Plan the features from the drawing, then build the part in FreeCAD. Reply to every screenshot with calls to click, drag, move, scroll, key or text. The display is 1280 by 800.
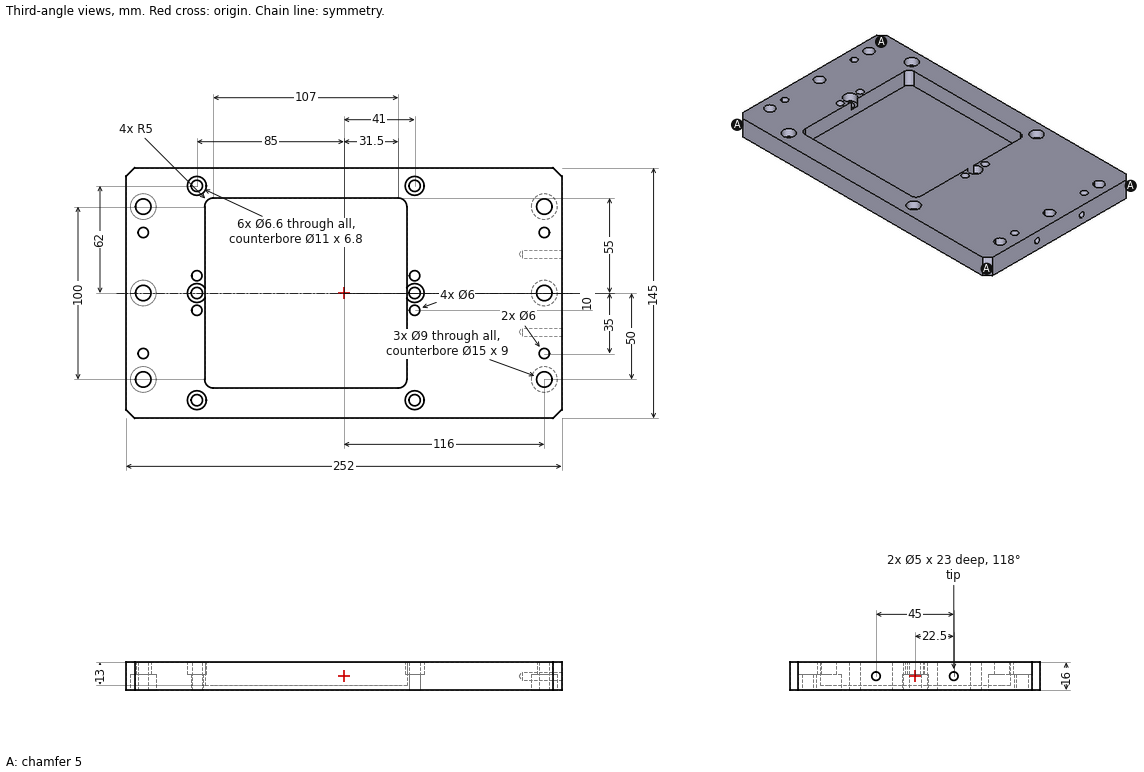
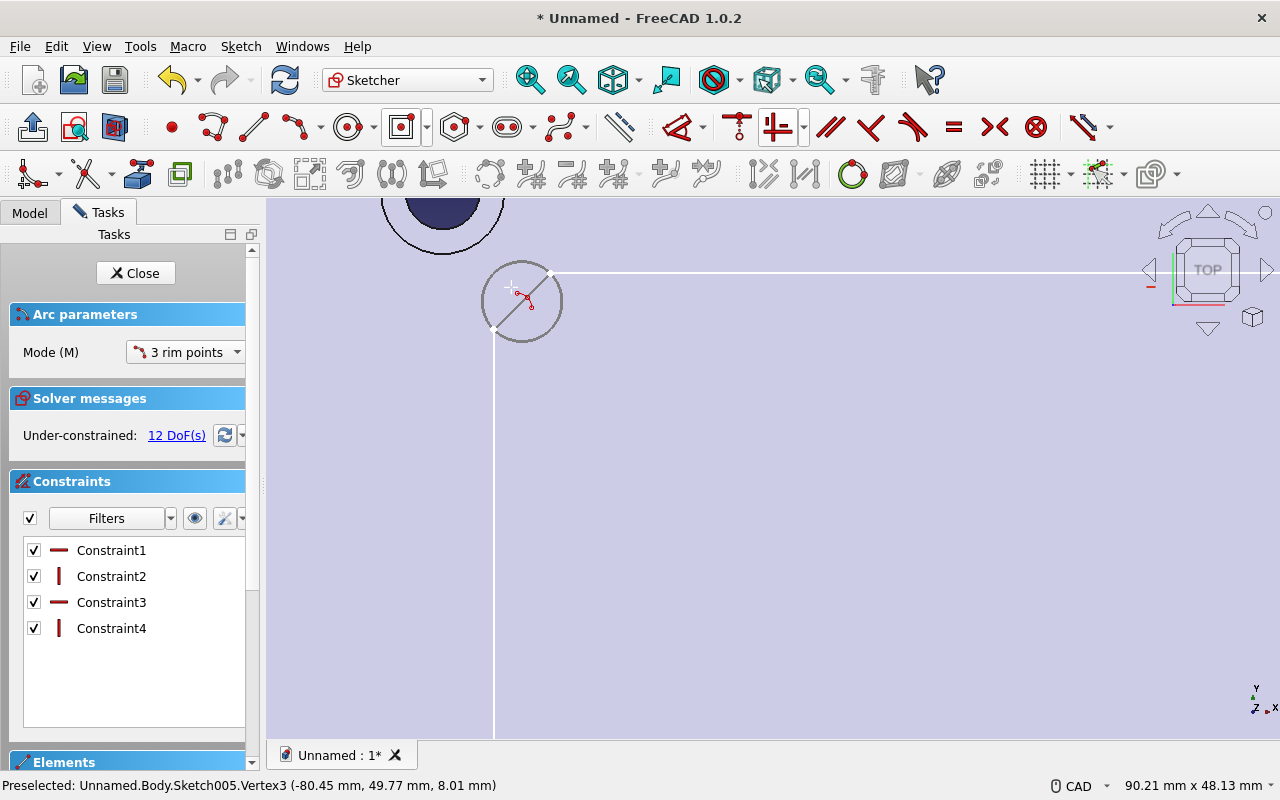
click(510, 287)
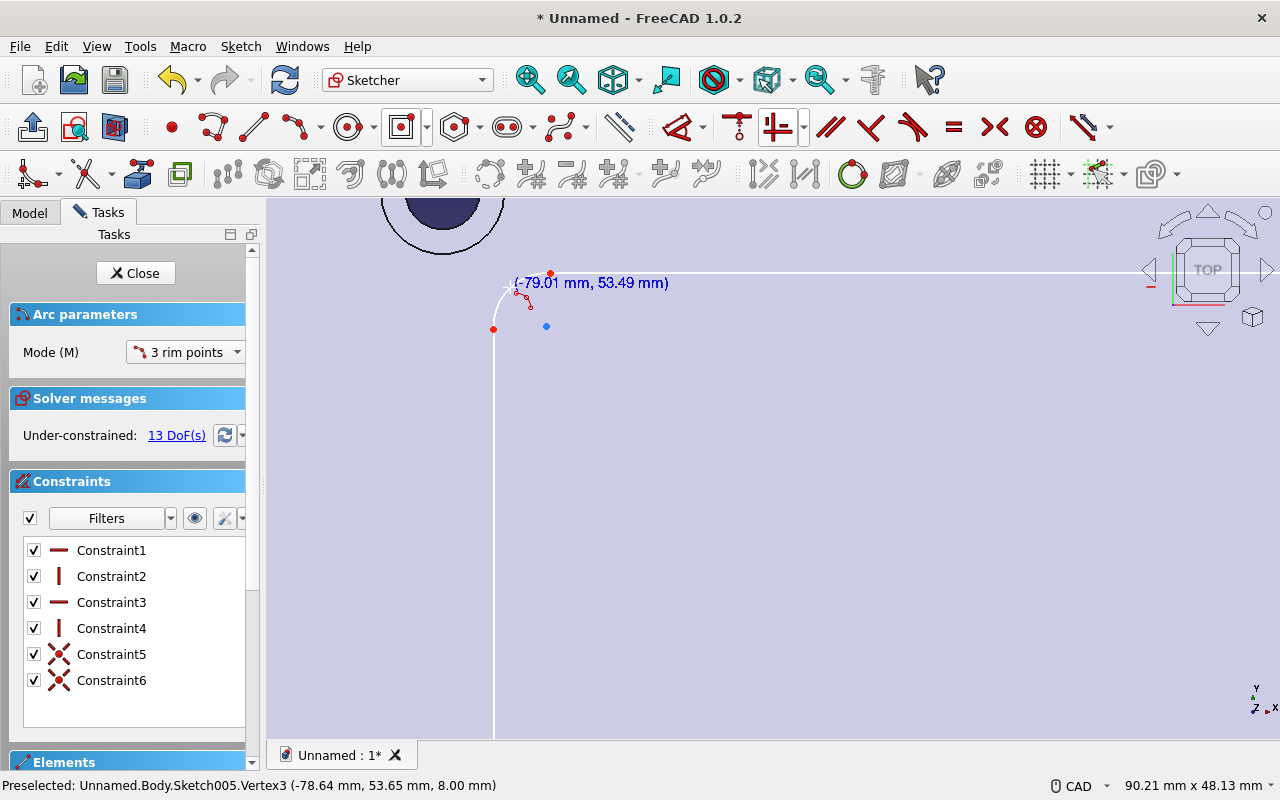
scroll(512, 287, down, 6)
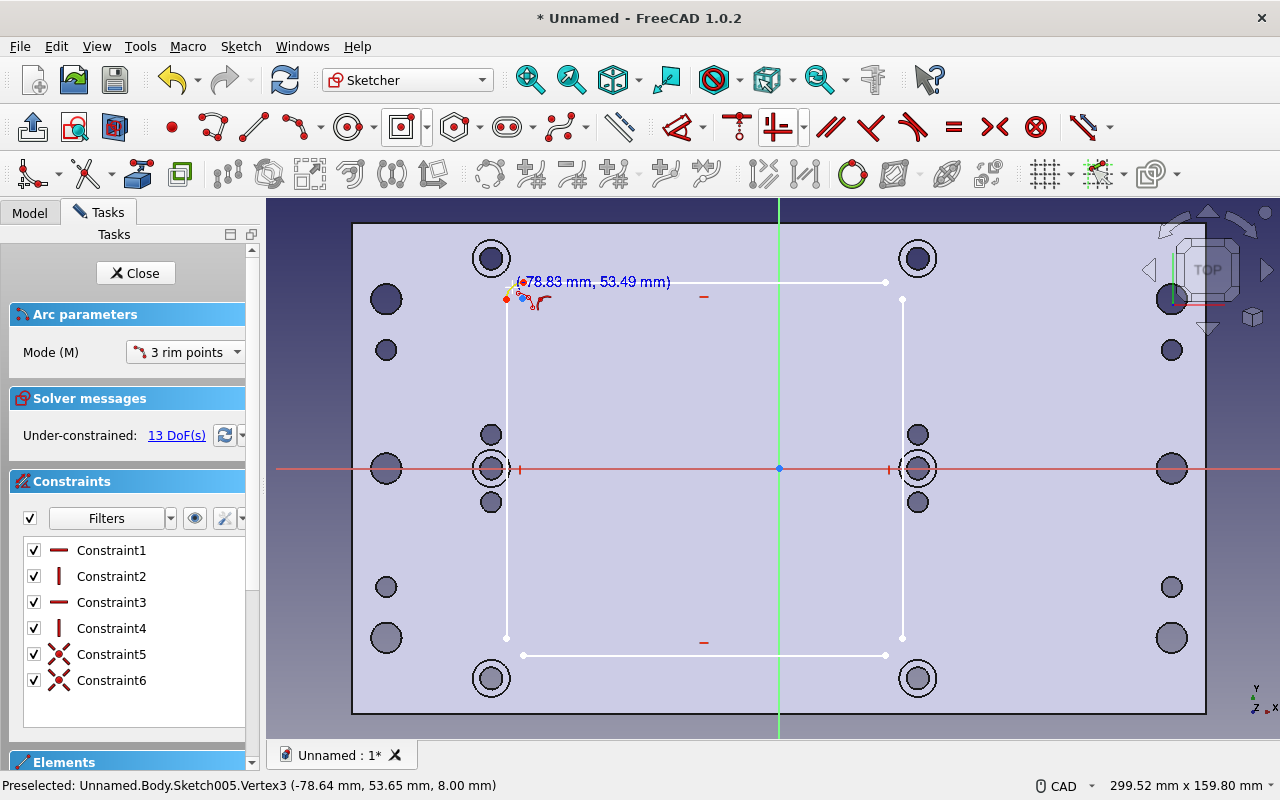
click(507, 639)
click(524, 656)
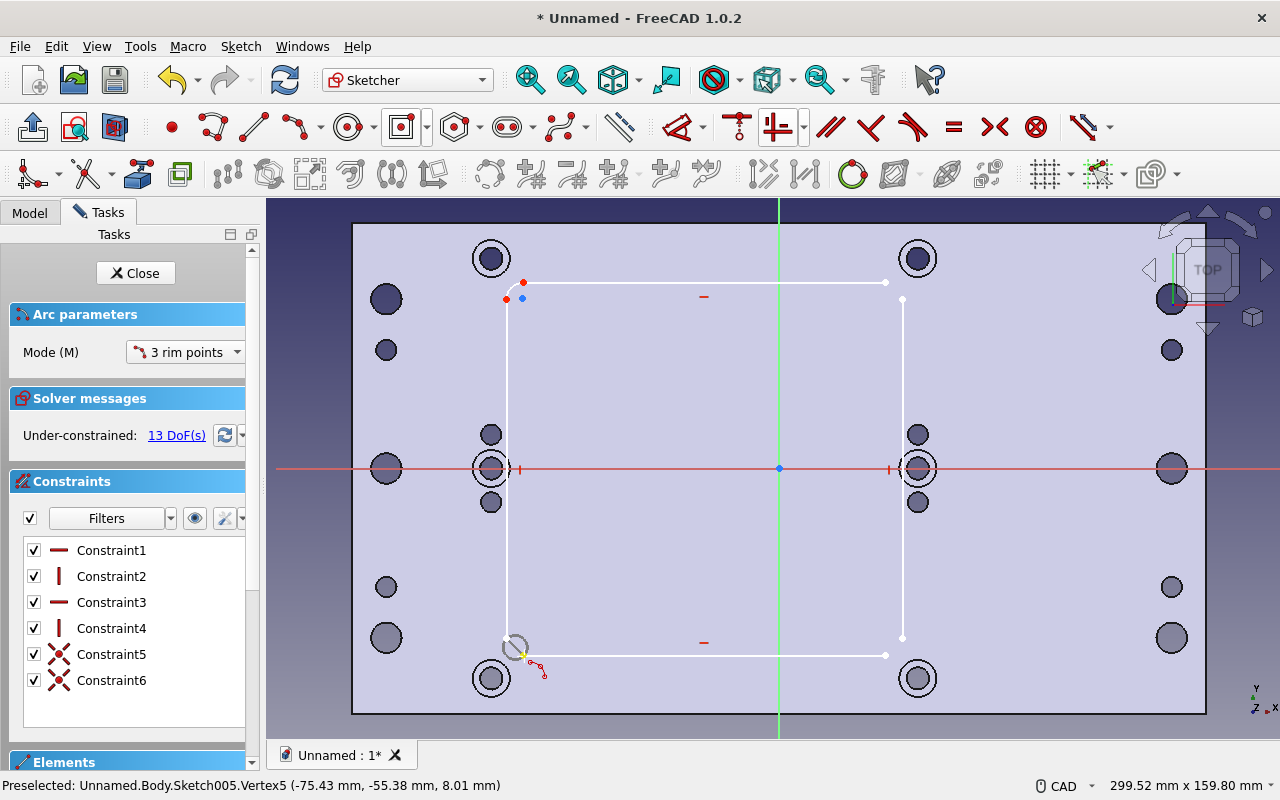
scroll(511, 650, up, 6)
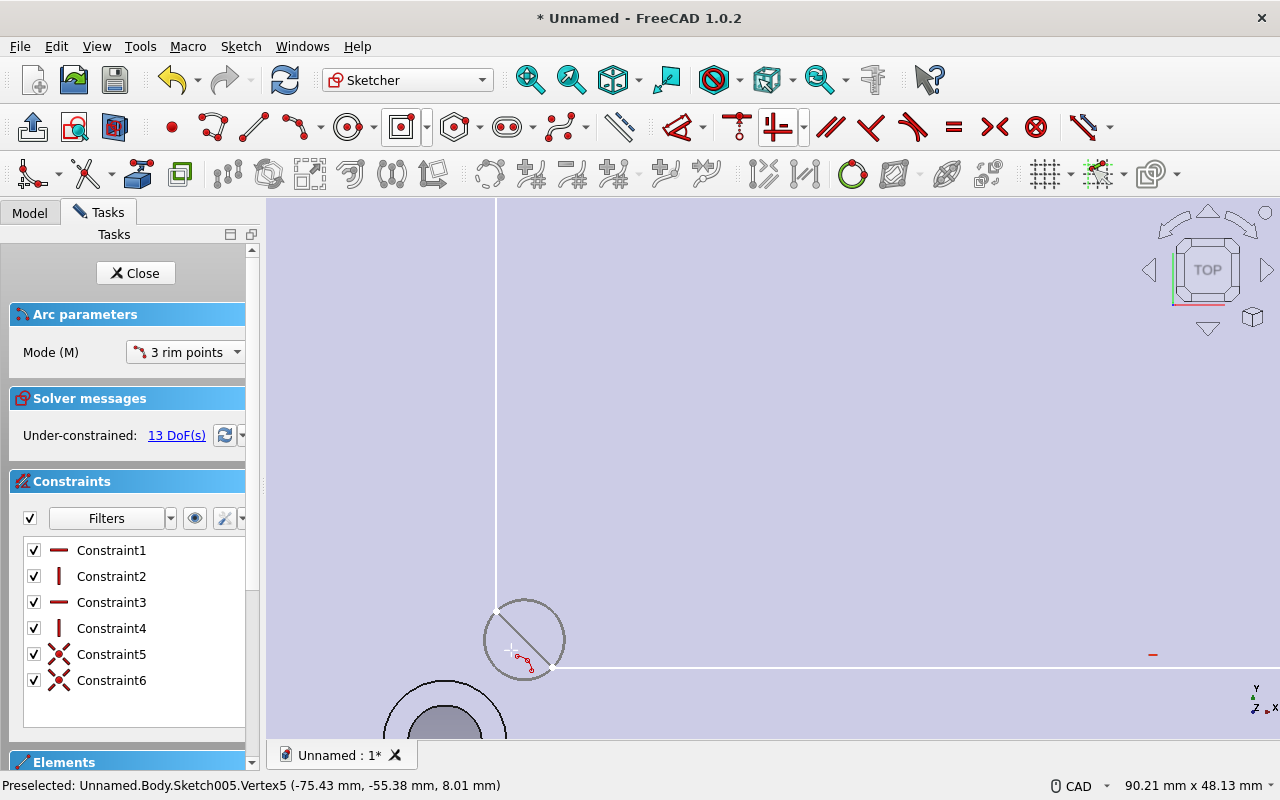
click(512, 647)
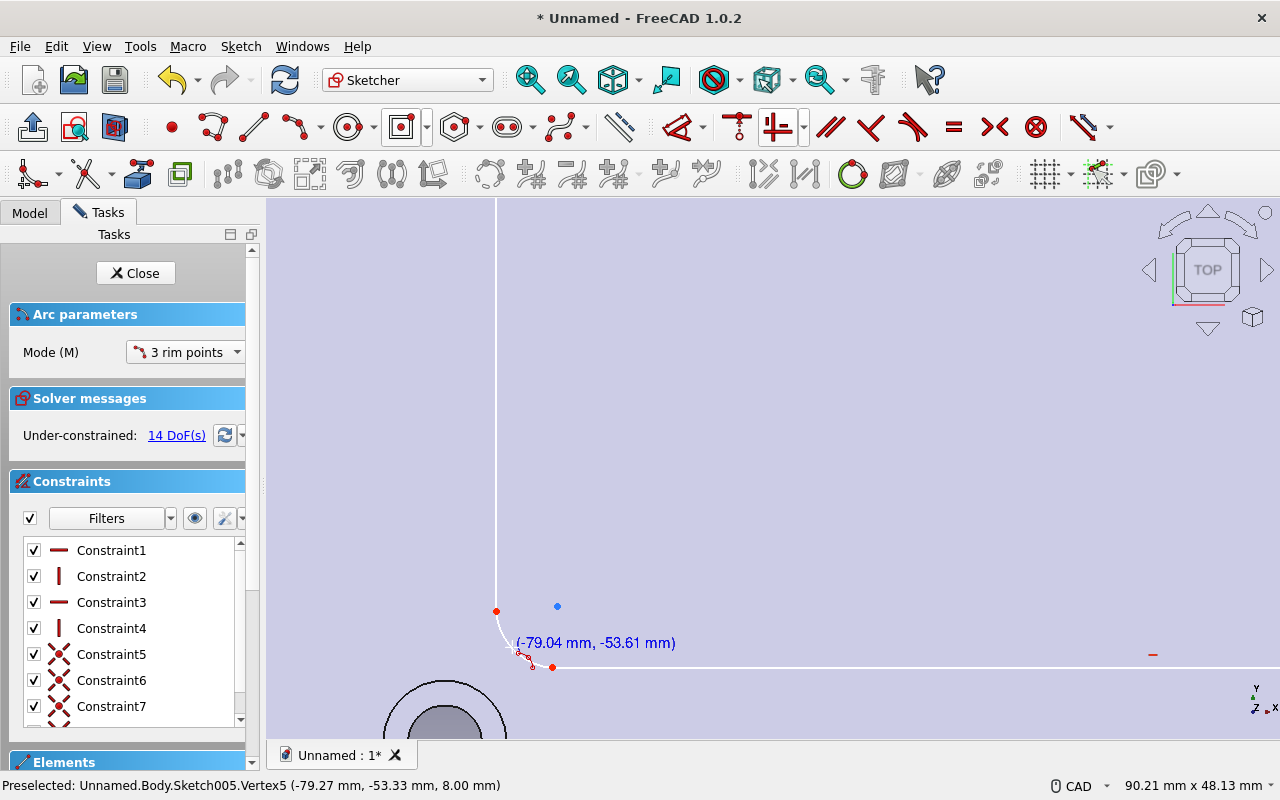
scroll(511, 651, down, 6)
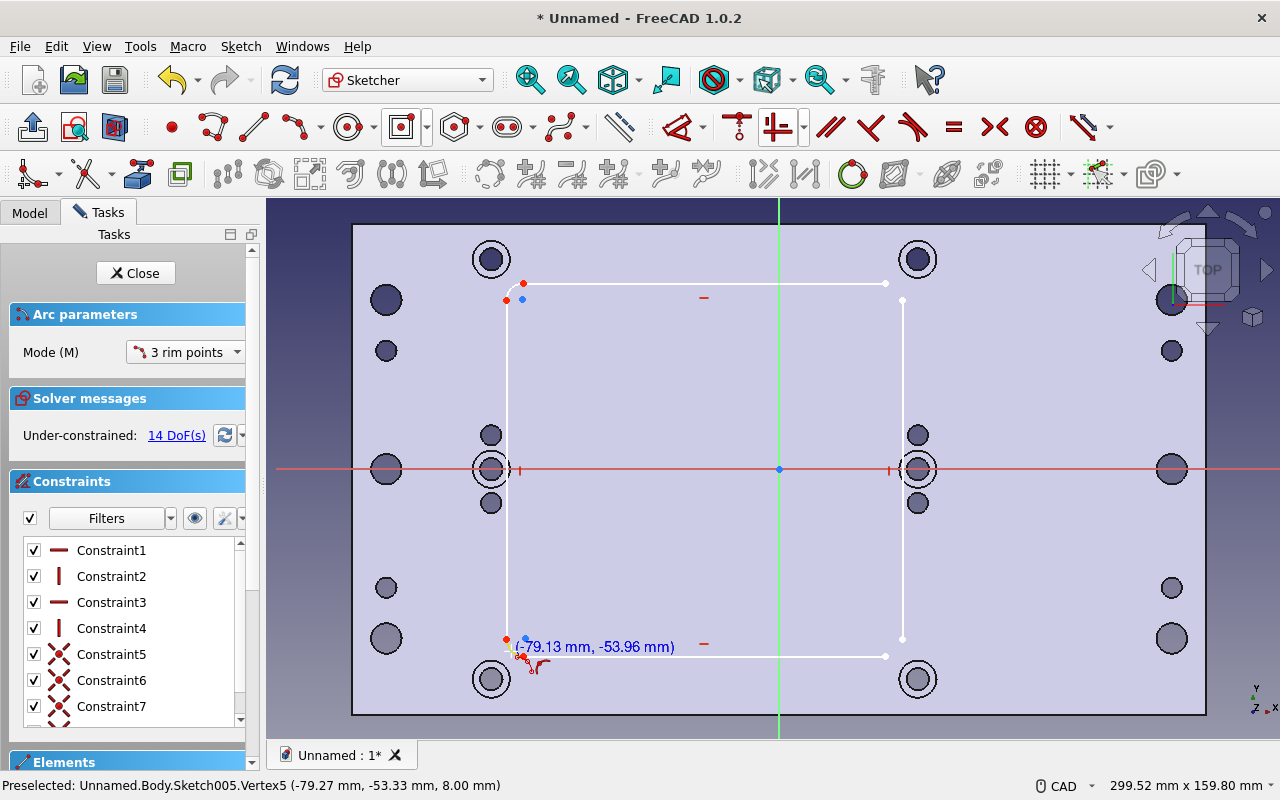
click(886, 657)
click(903, 640)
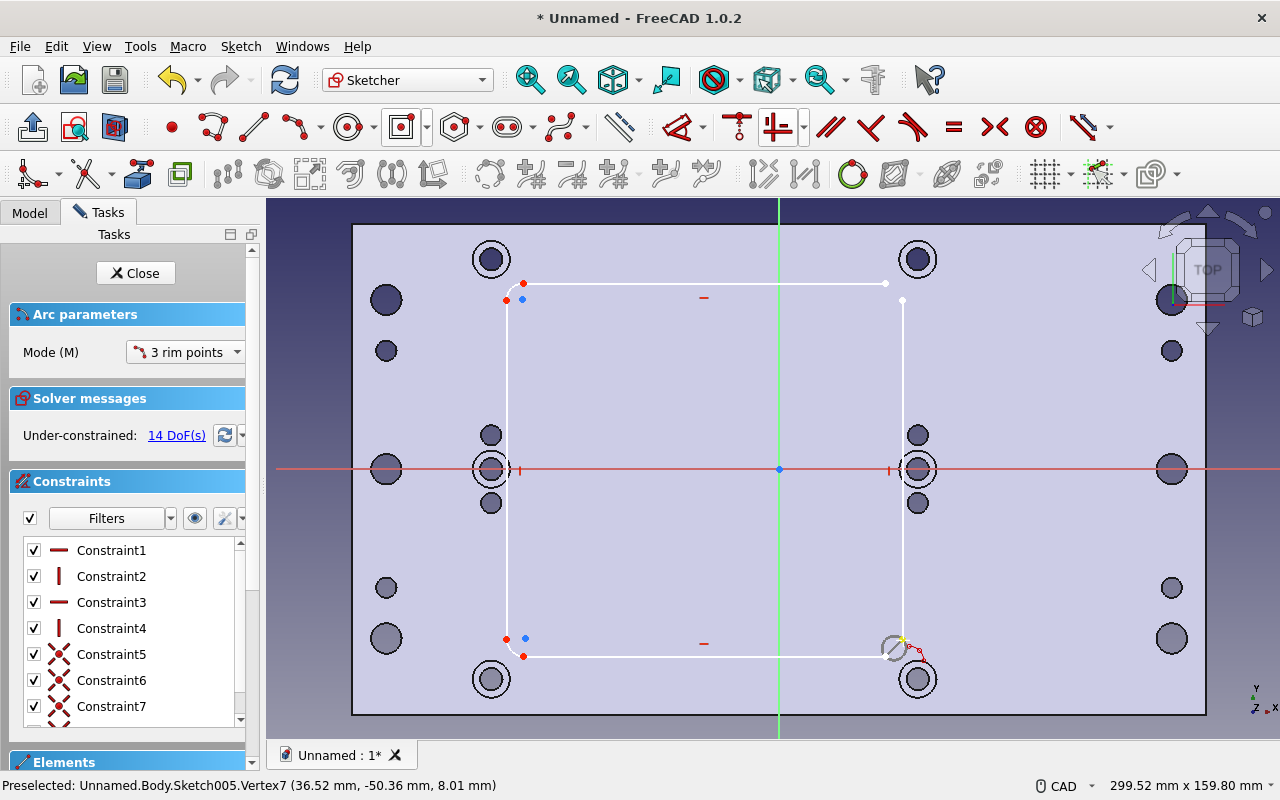
scroll(898, 650, up, 6)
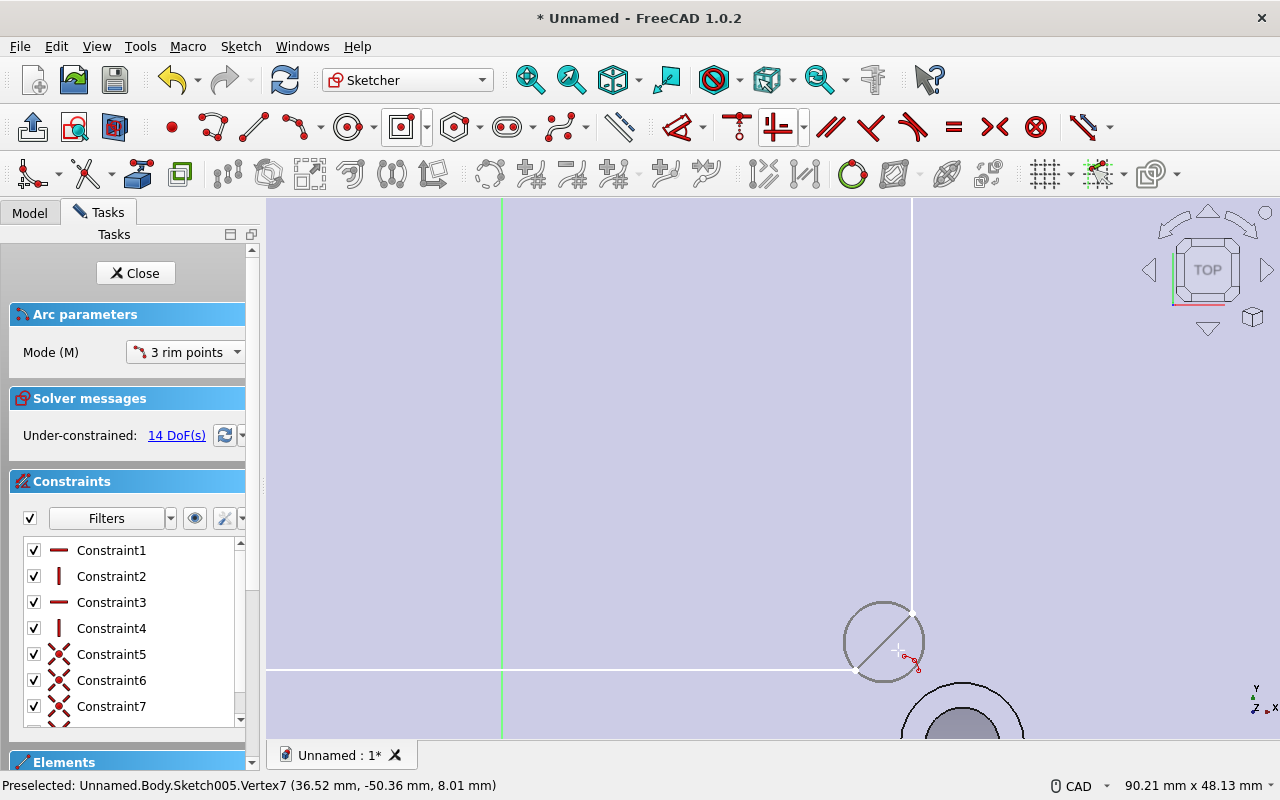
click(895, 650)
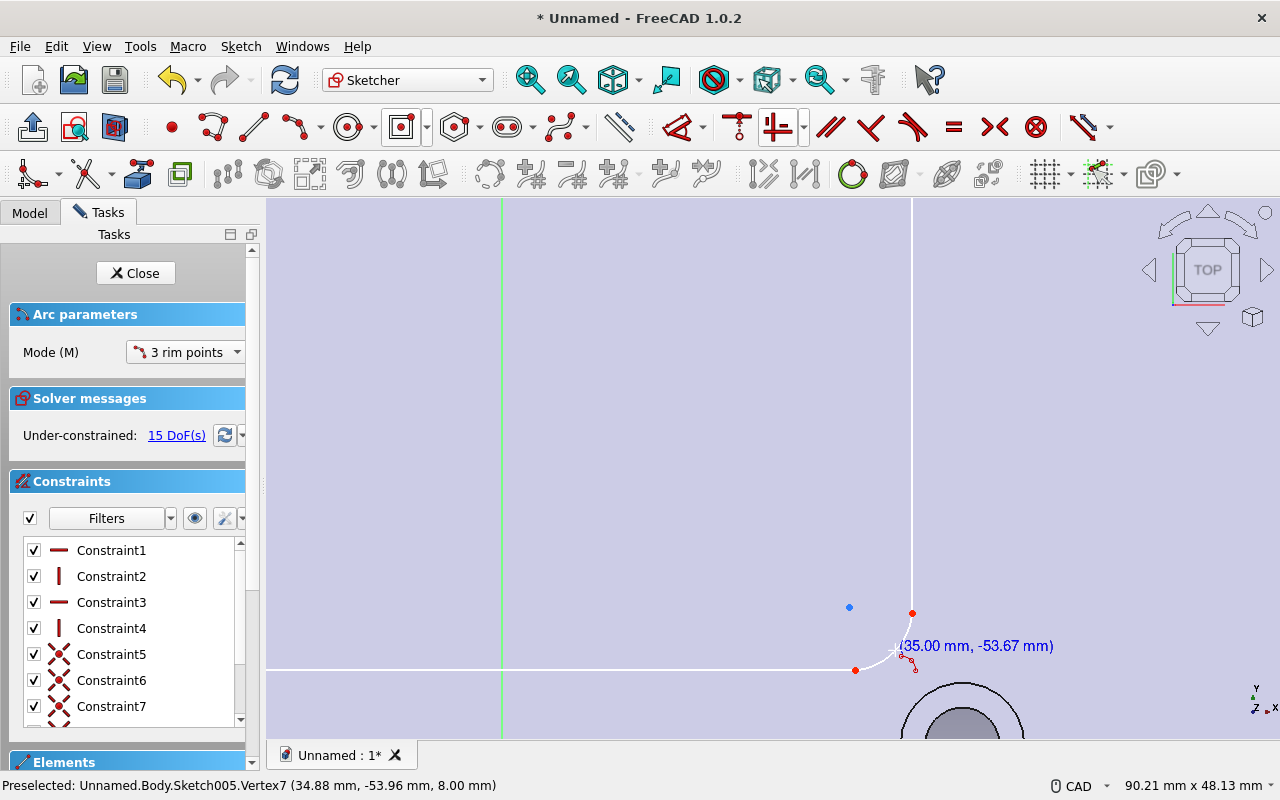
scroll(899, 650, down, 6)